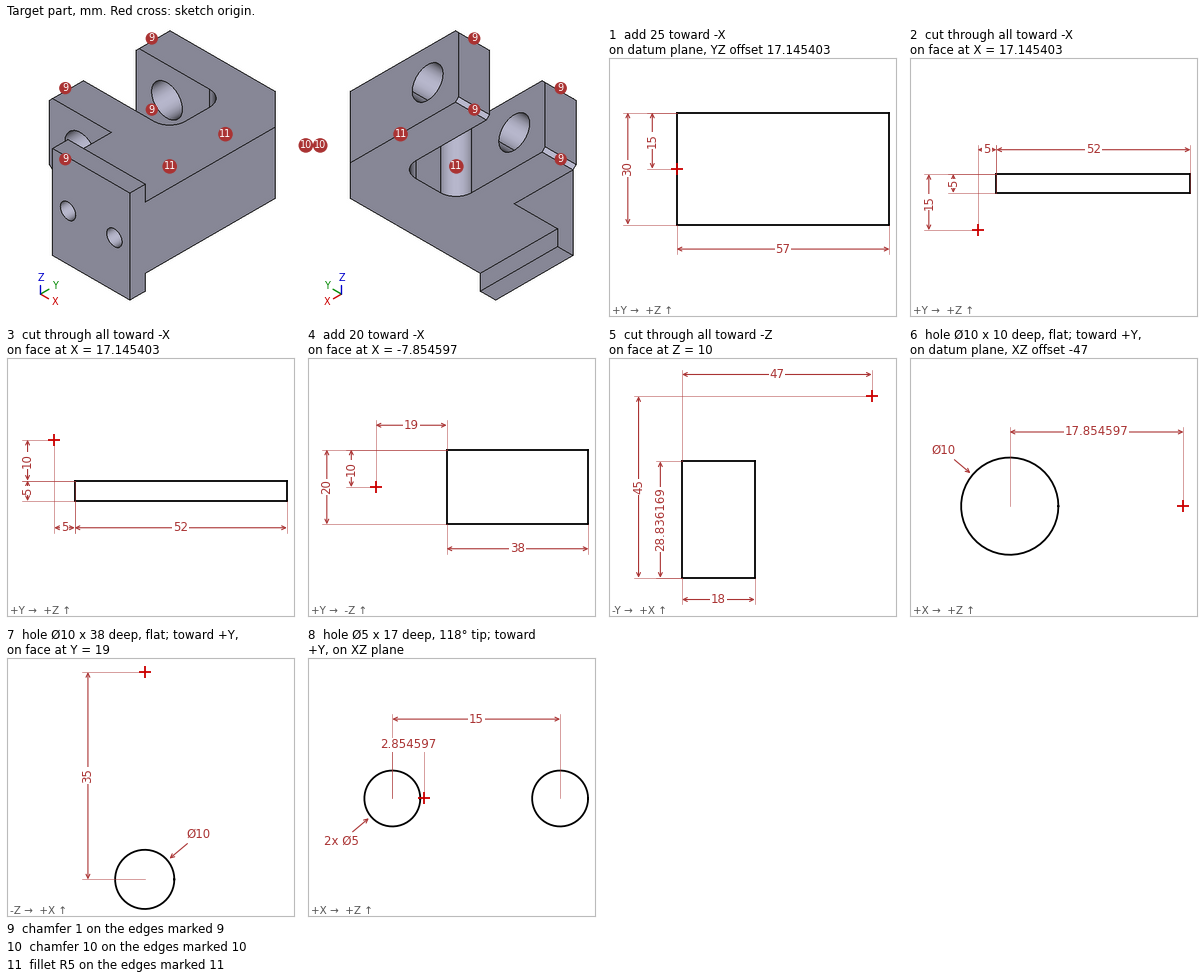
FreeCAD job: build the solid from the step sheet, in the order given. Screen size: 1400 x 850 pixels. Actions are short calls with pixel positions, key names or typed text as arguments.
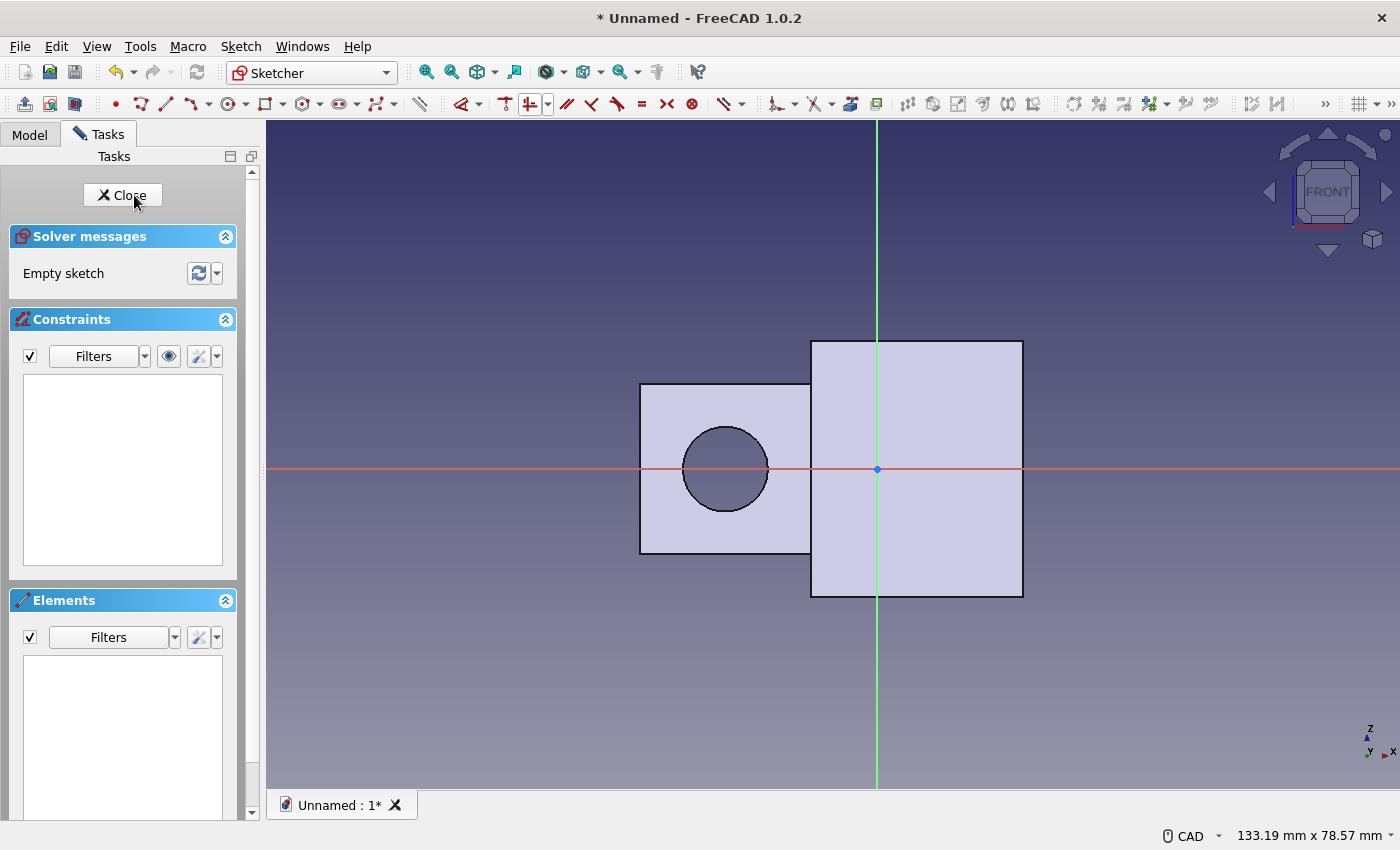
scroll(967, 474, up, 7)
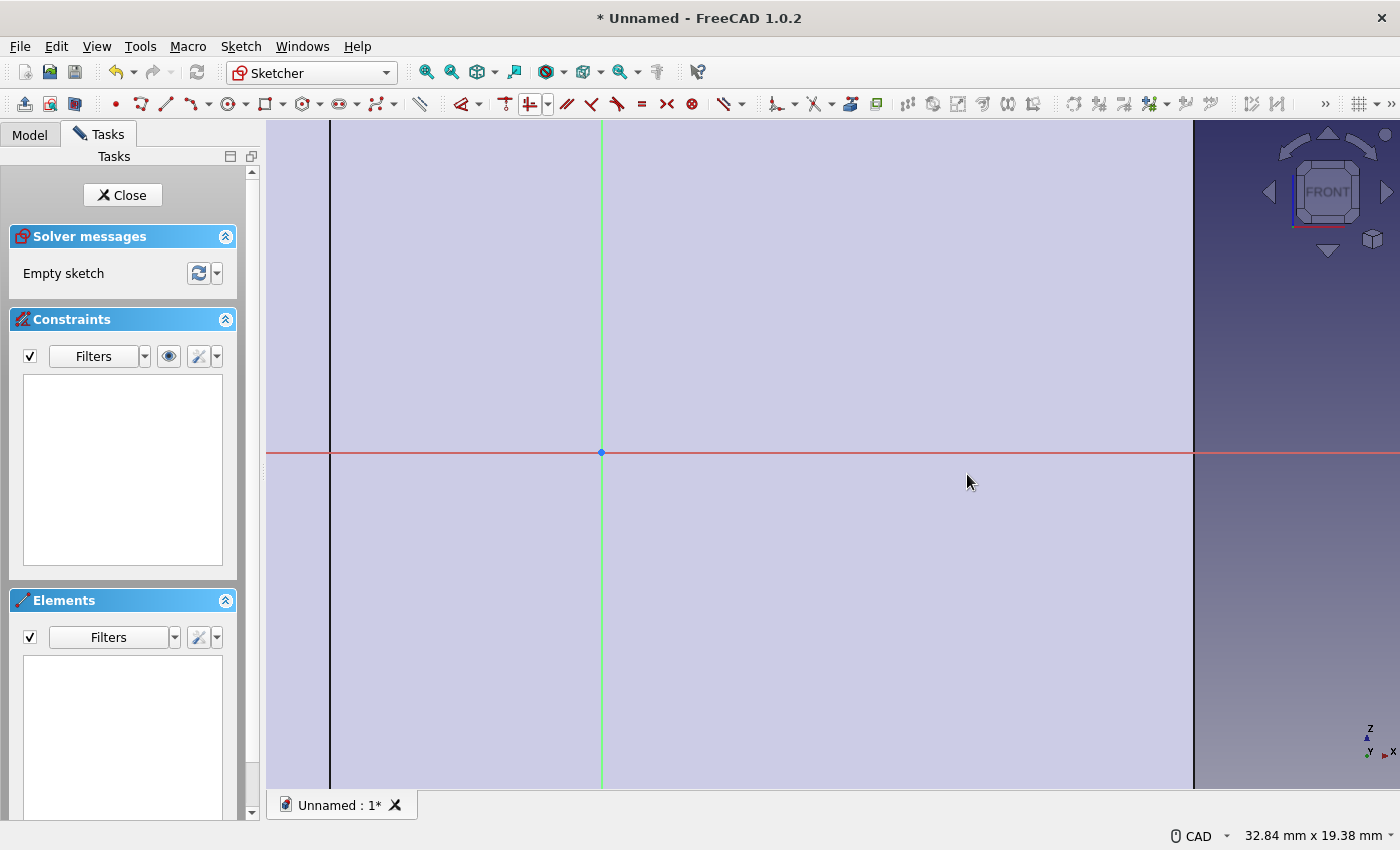
click(228, 104)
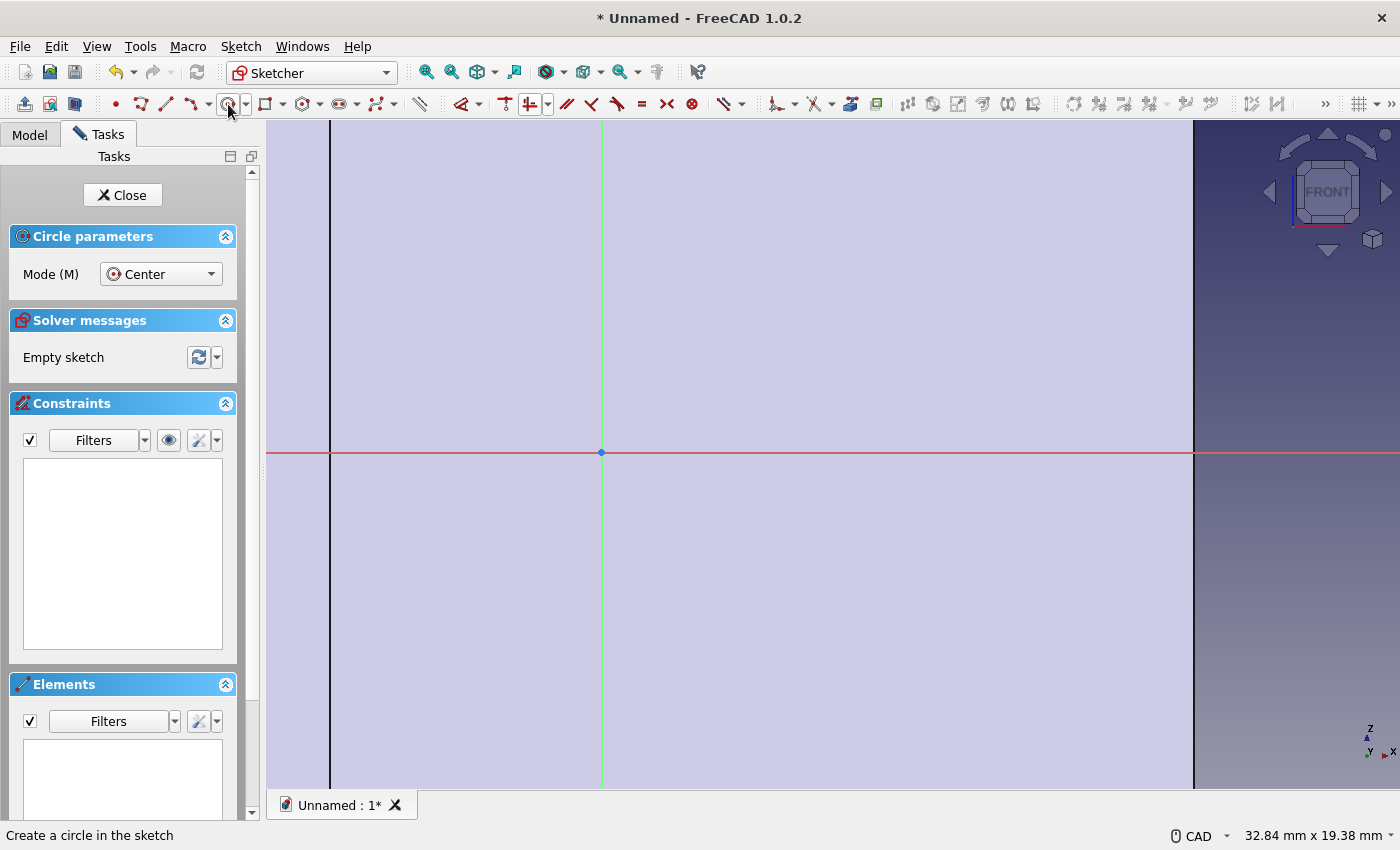
click(503, 453)
click(564, 392)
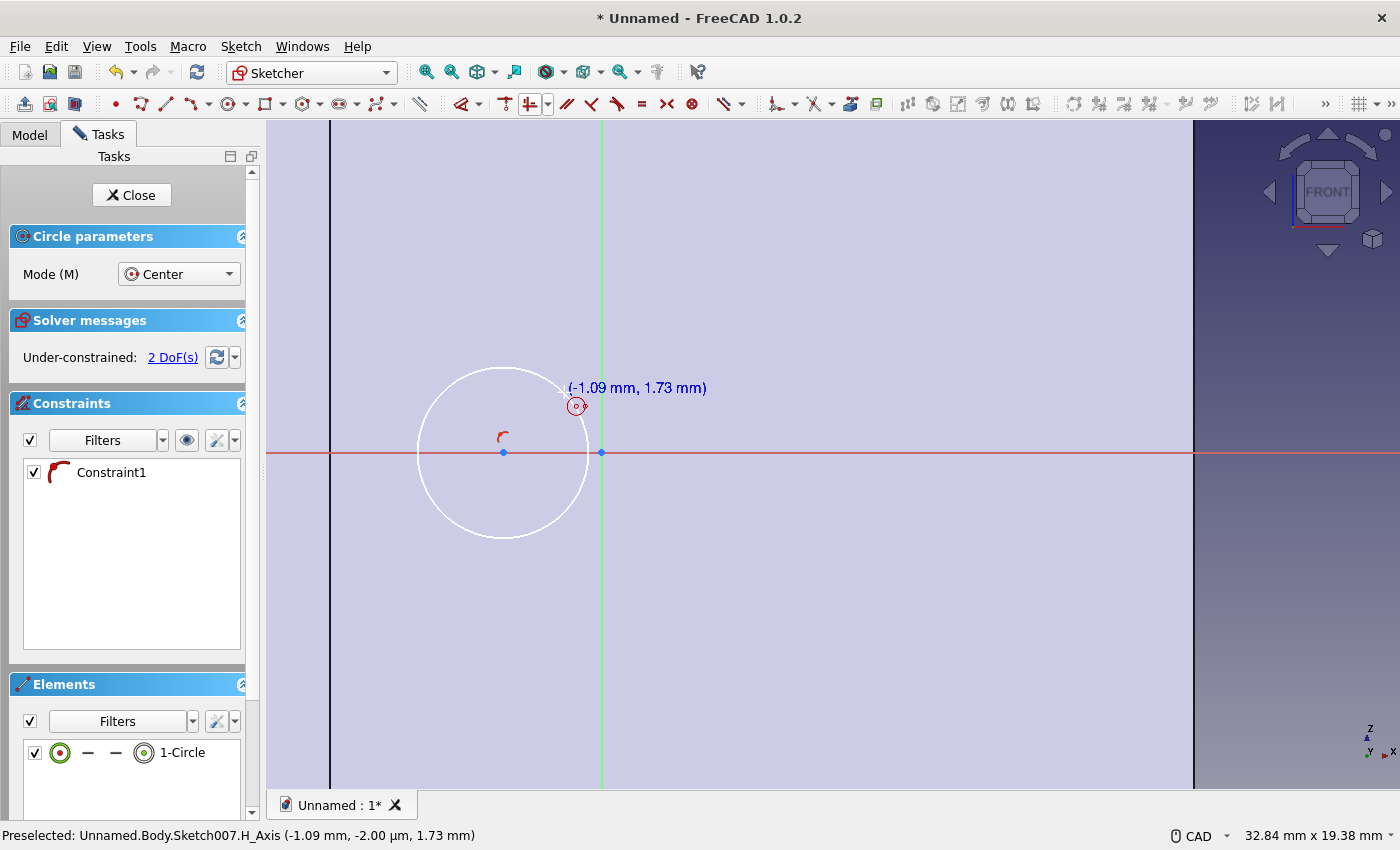
click(1021, 453)
click(1082, 392)
key(Escape)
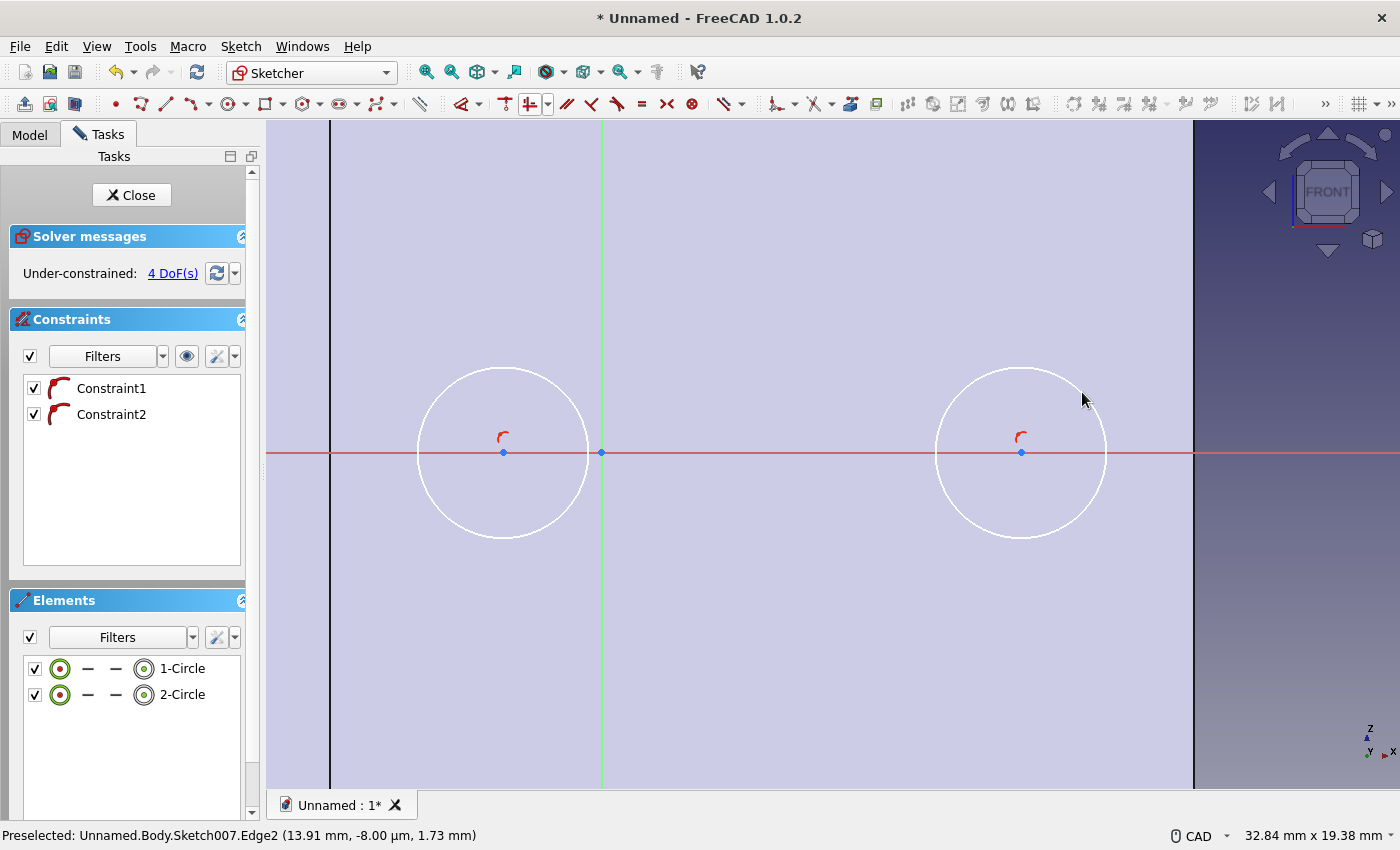
click(563, 392)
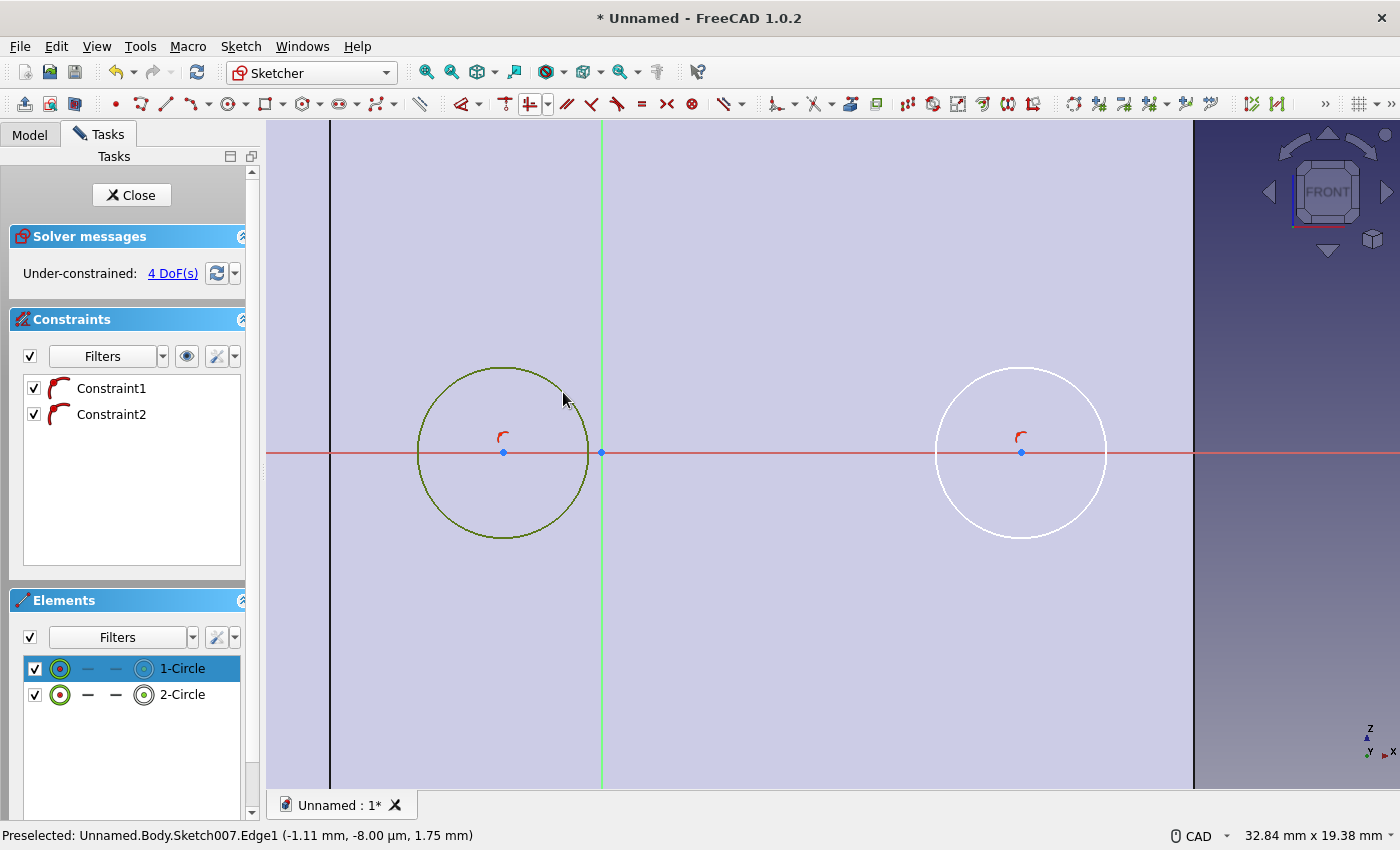
click(1081, 392)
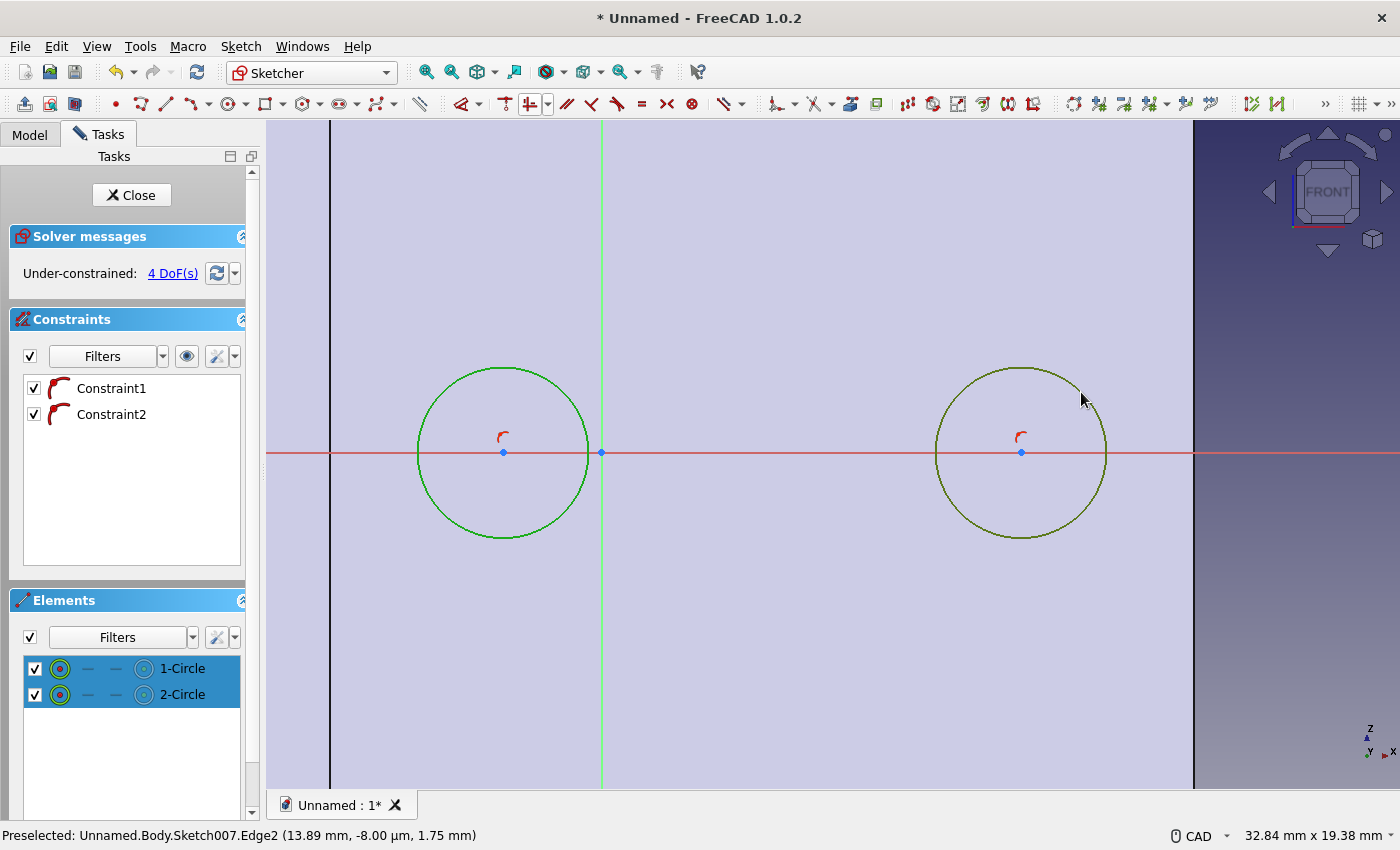
key(e)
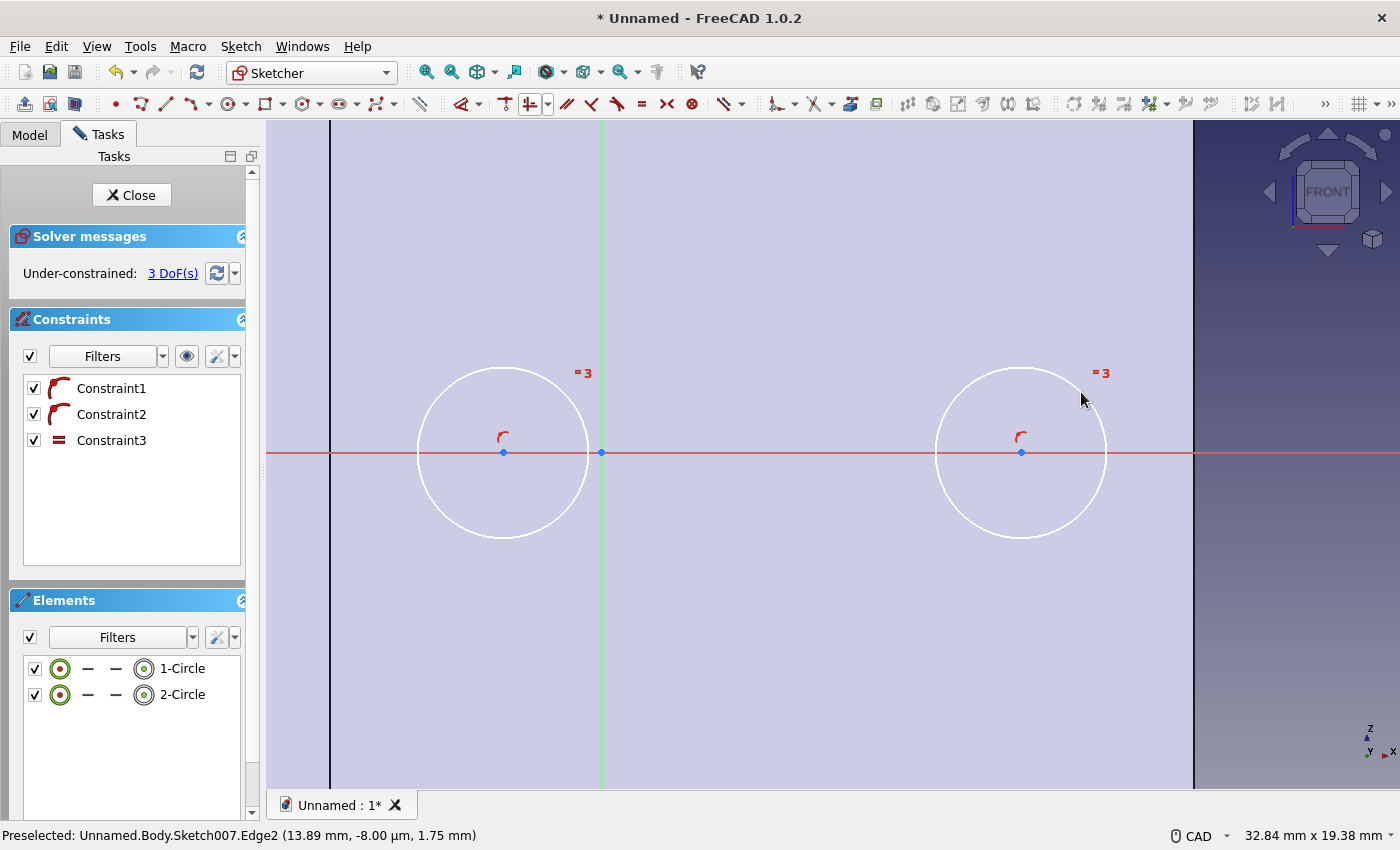
click(460, 104)